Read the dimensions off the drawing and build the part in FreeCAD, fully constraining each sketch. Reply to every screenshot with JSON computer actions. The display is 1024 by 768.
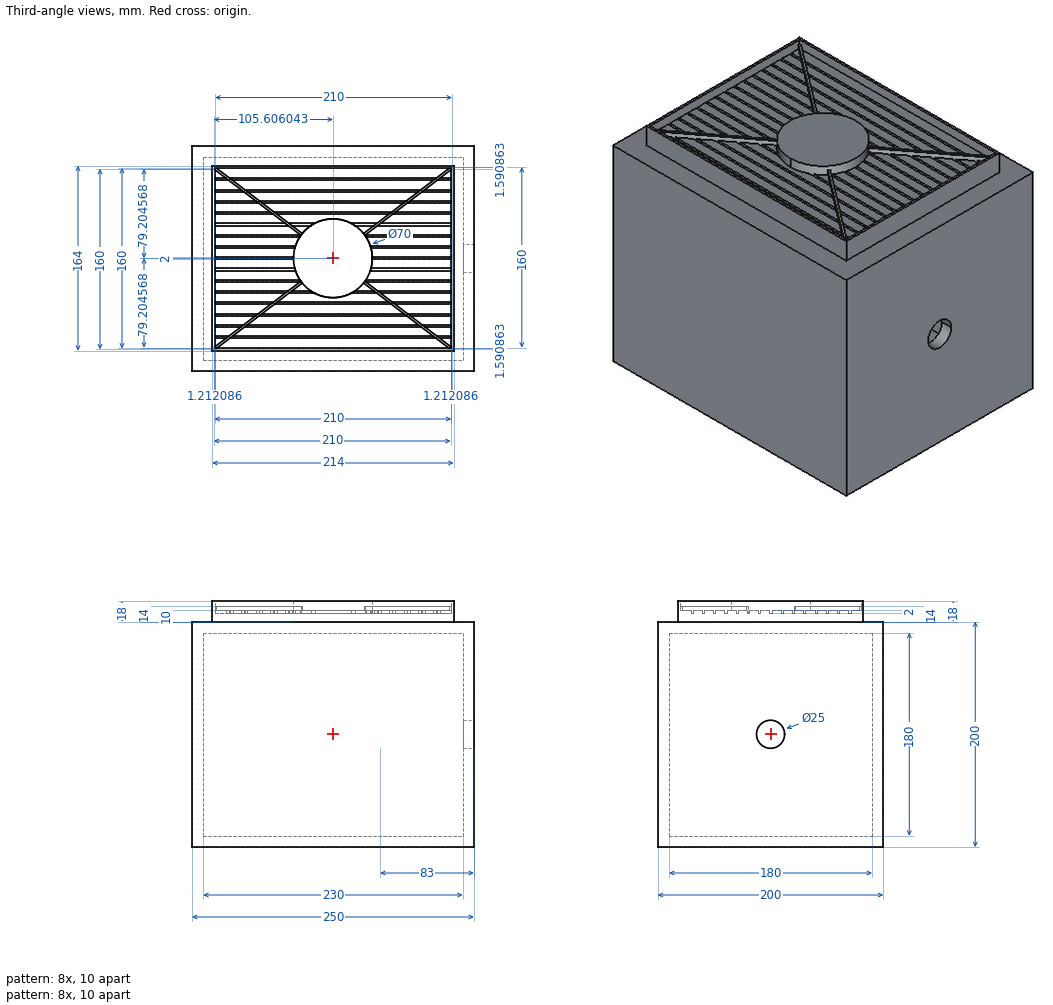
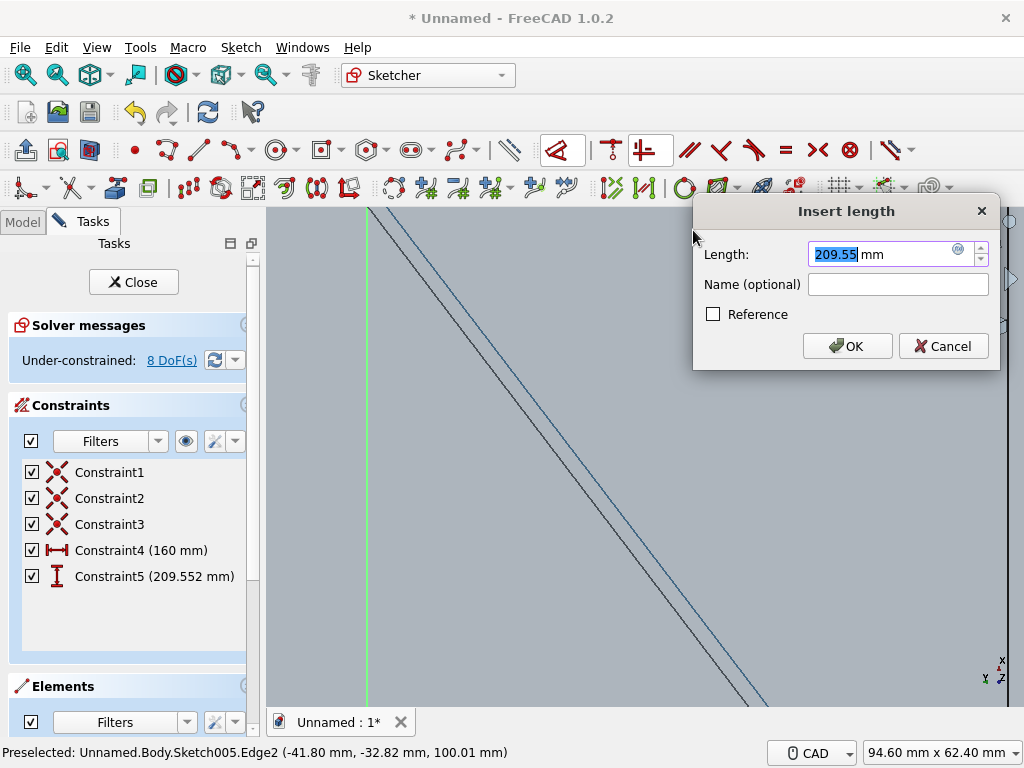
{"action": "type", "text": "210"}
{"action": "key", "text": "Return"}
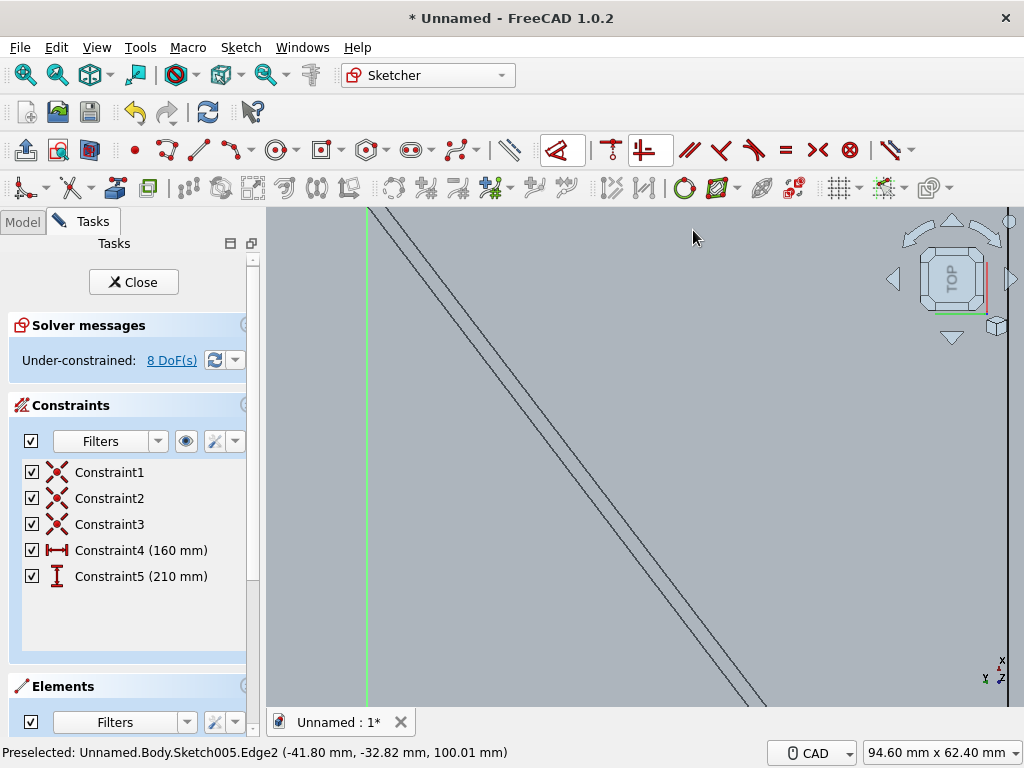
{"action": "left_click", "coordinate": [617, 534]}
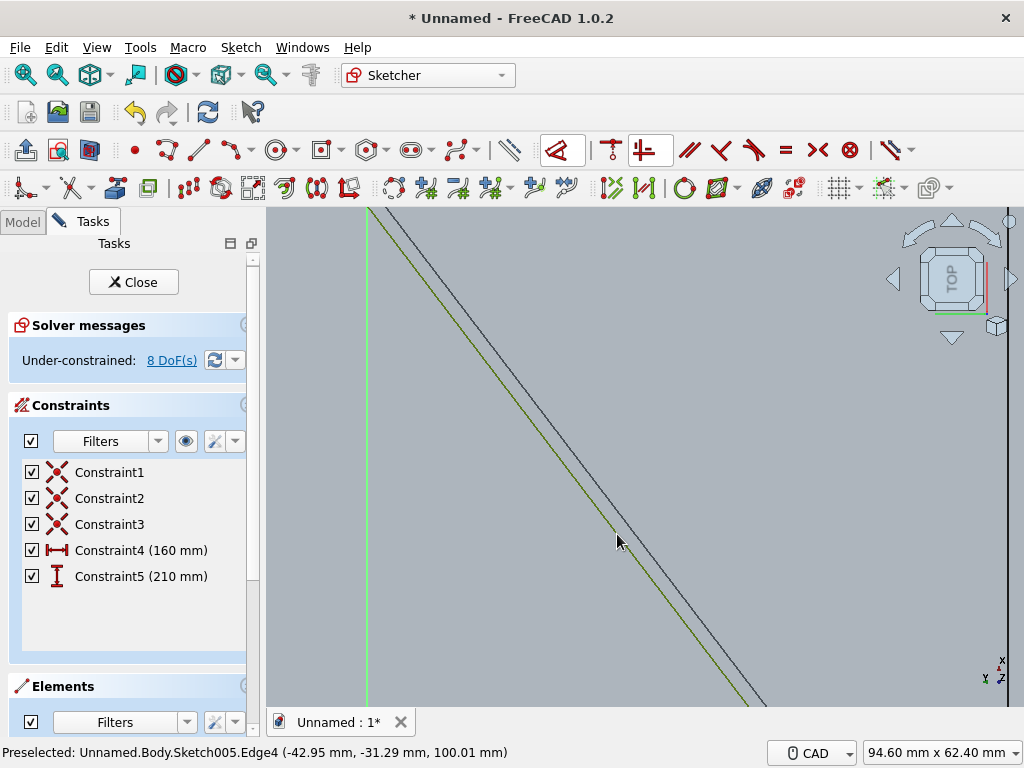
{"action": "key", "text": "l"}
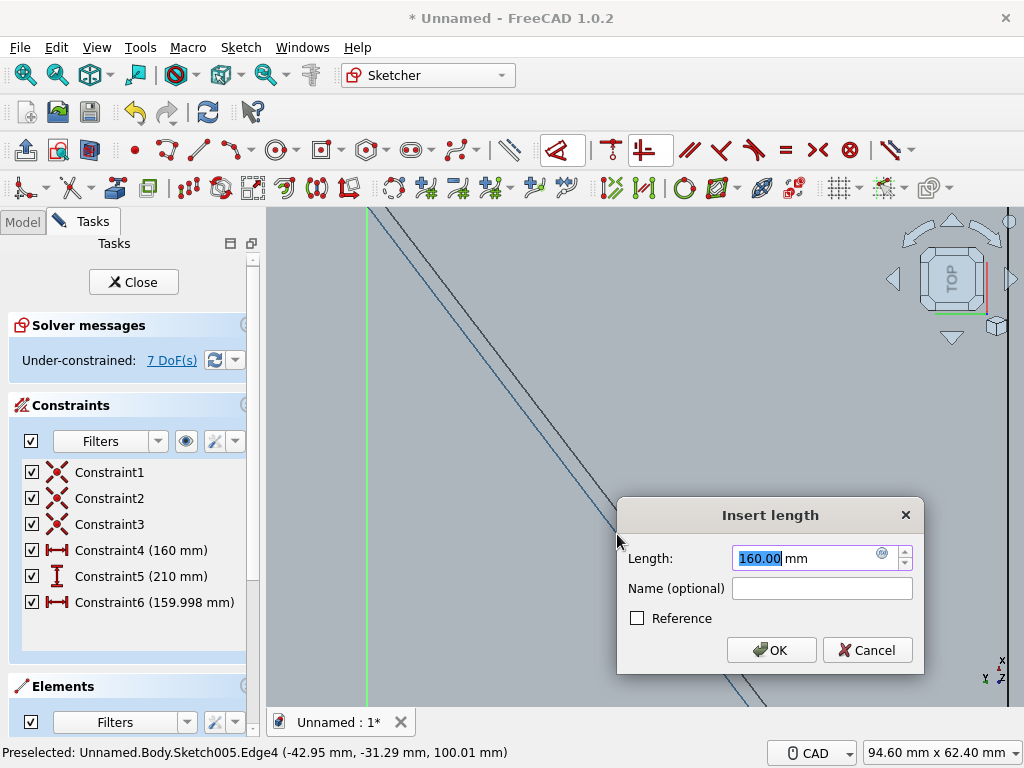
{"action": "type", "text": "160"}
{"action": "key", "text": "Return"}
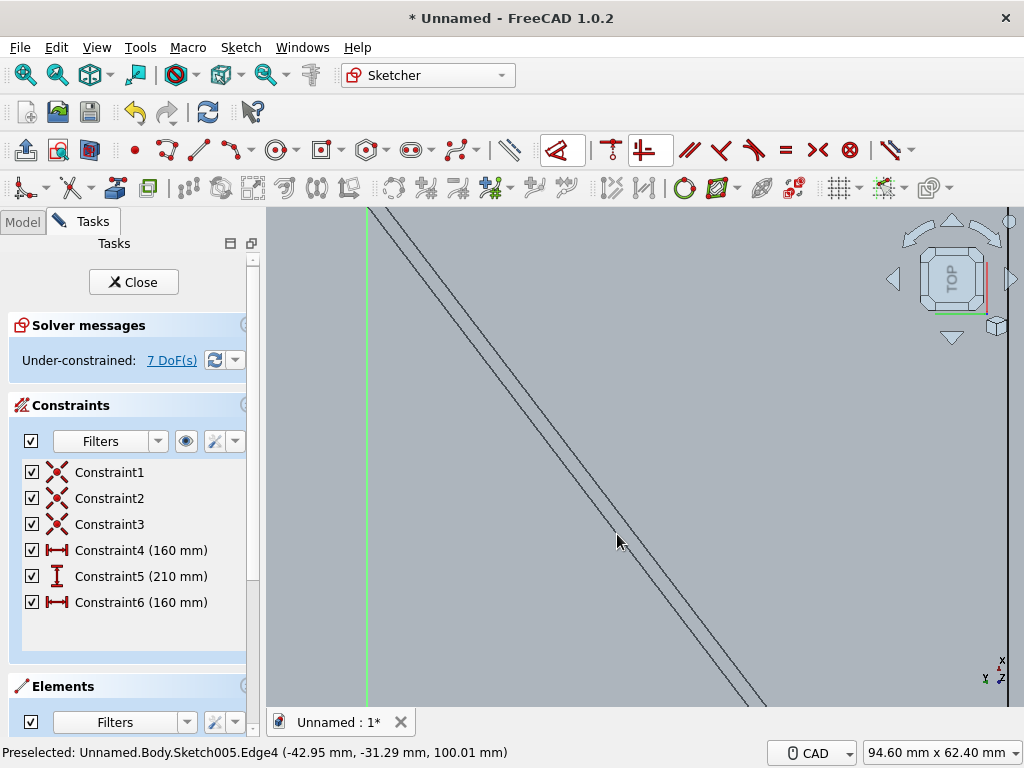
{"action": "left_click", "coordinate": [617, 534]}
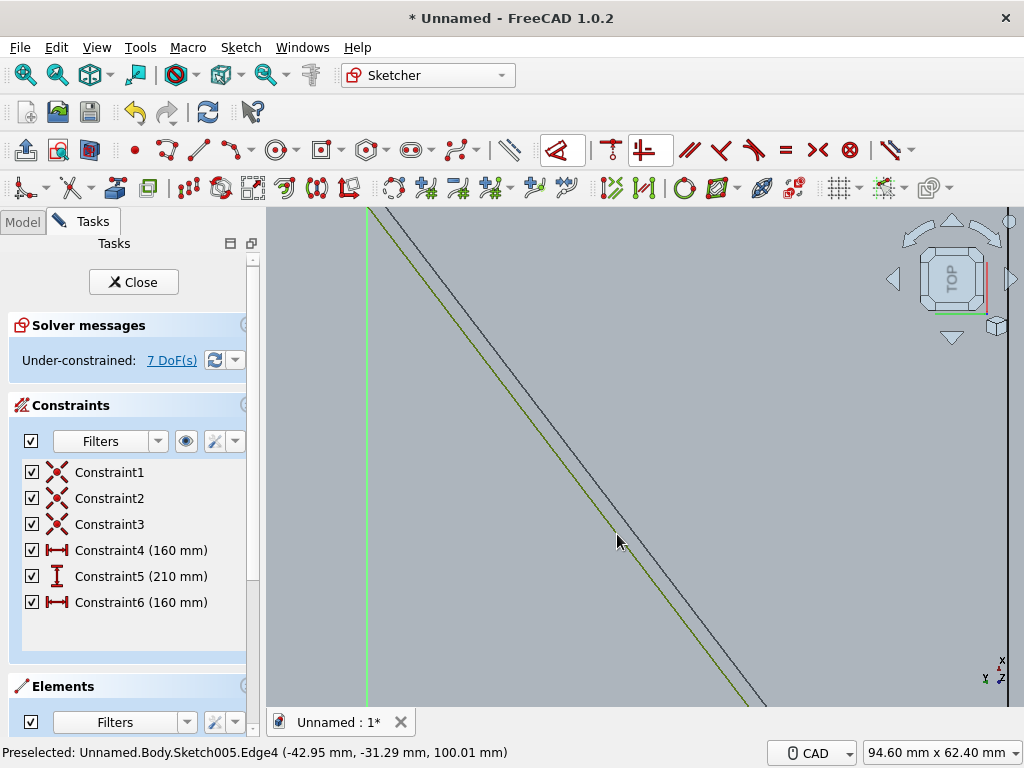
{"action": "left_click", "coordinate": [580, 150]}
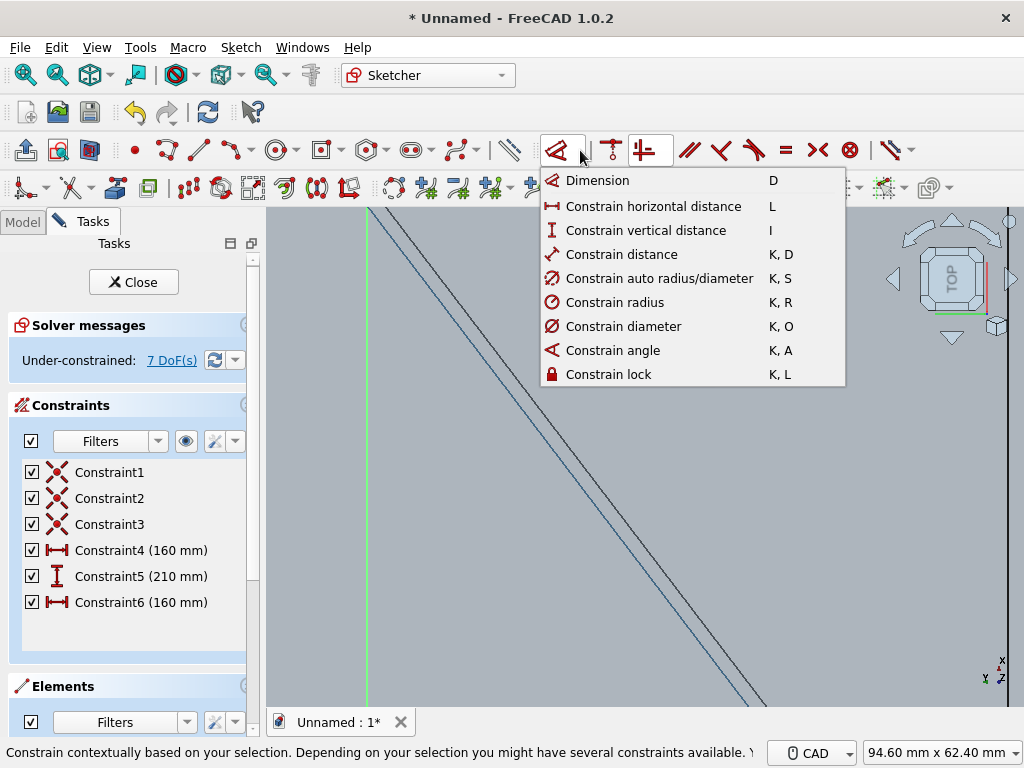
{"action": "left_click", "coordinate": [693, 230]}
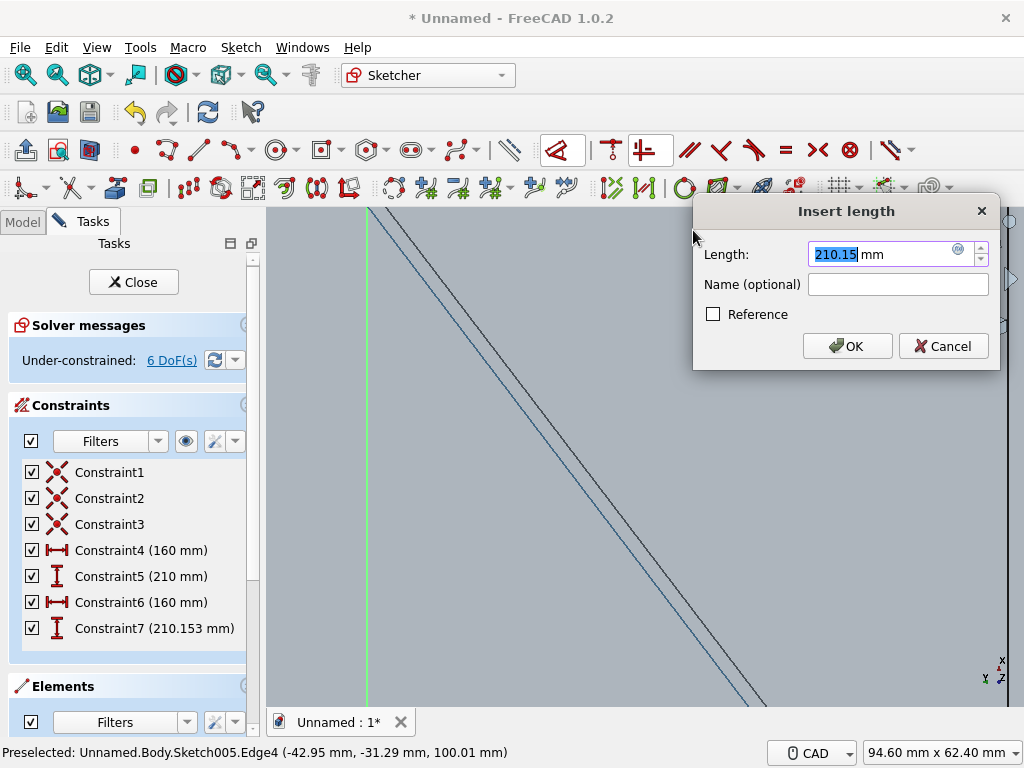
{"action": "type", "text": "210"}
{"action": "key", "text": "Return"}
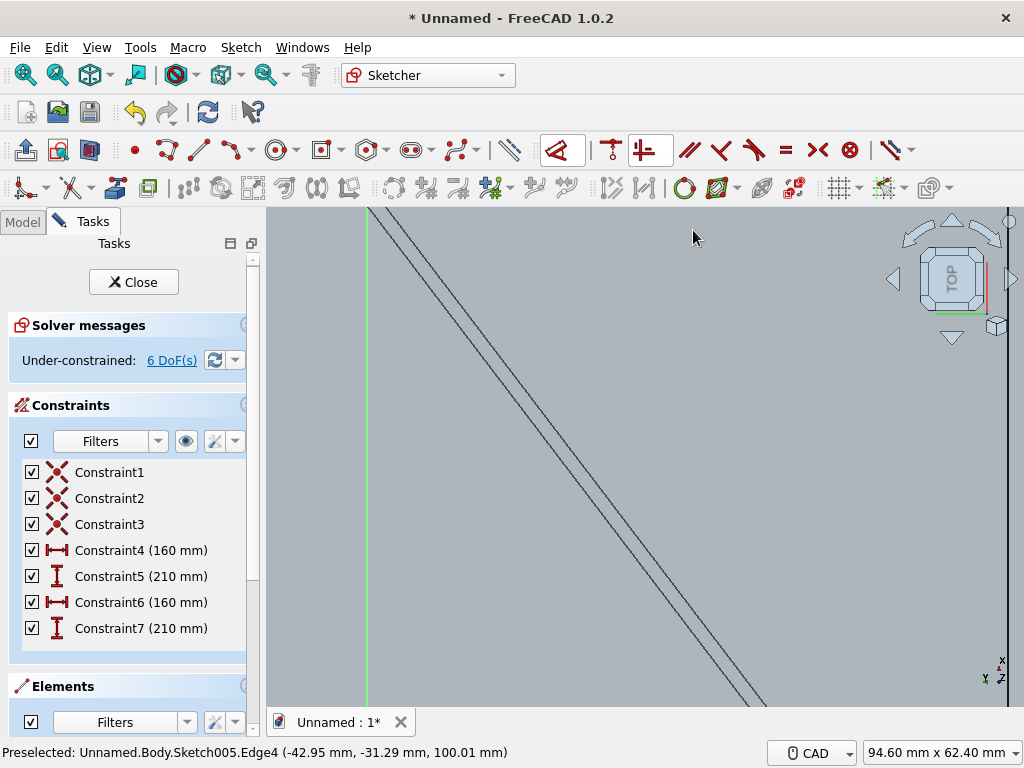
{"action": "scroll", "coordinate": [630, 524], "scroll_direction": "down", "scroll_amount": 8}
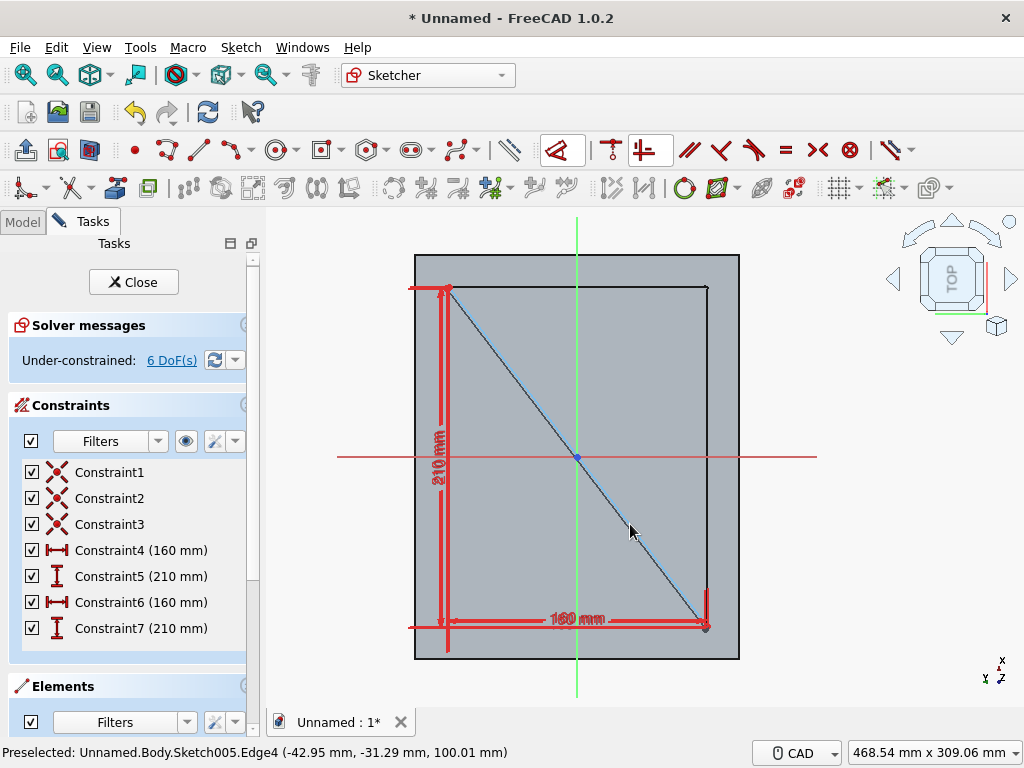
{"action": "scroll", "coordinate": [707, 628], "scroll_direction": "up", "scroll_amount": 14}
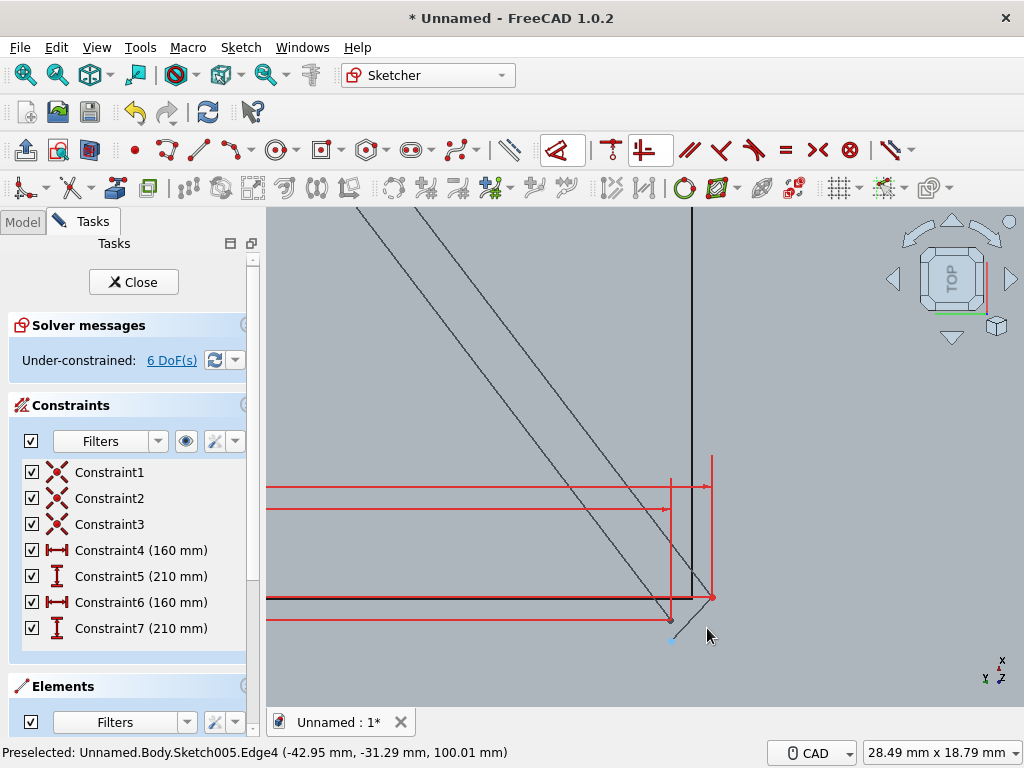
{"action": "left_click", "coordinate": [696, 615]}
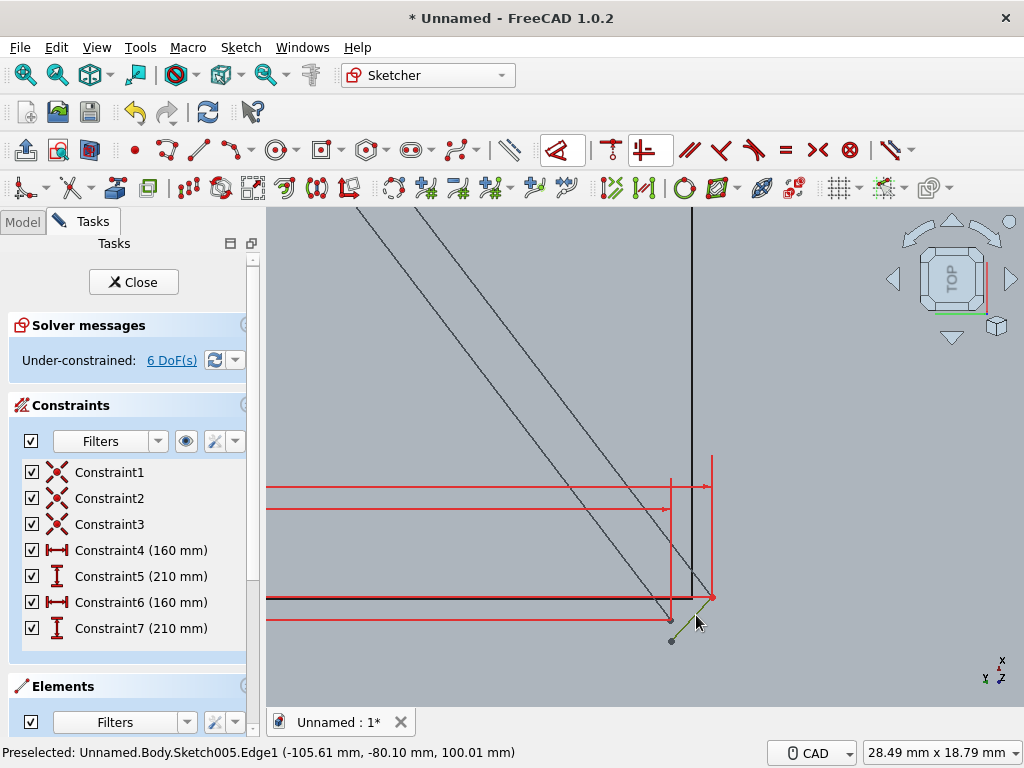
{"action": "key", "text": "l"}